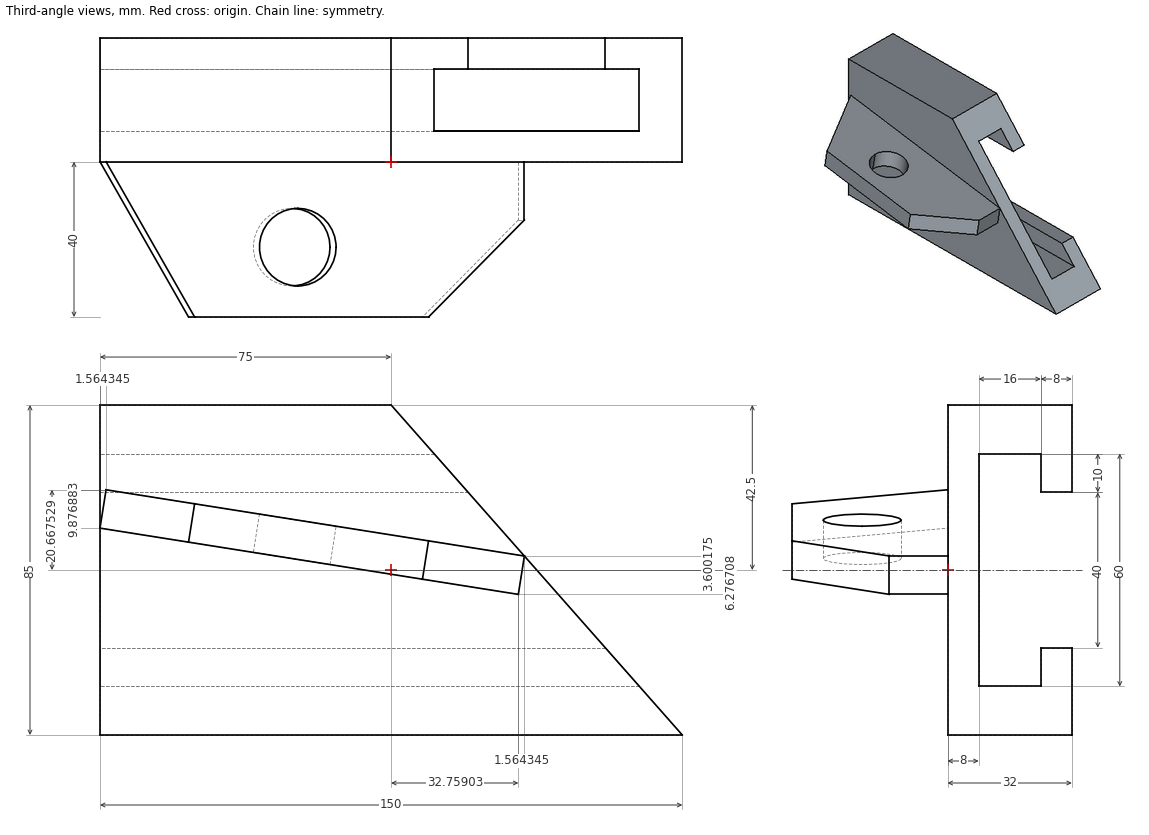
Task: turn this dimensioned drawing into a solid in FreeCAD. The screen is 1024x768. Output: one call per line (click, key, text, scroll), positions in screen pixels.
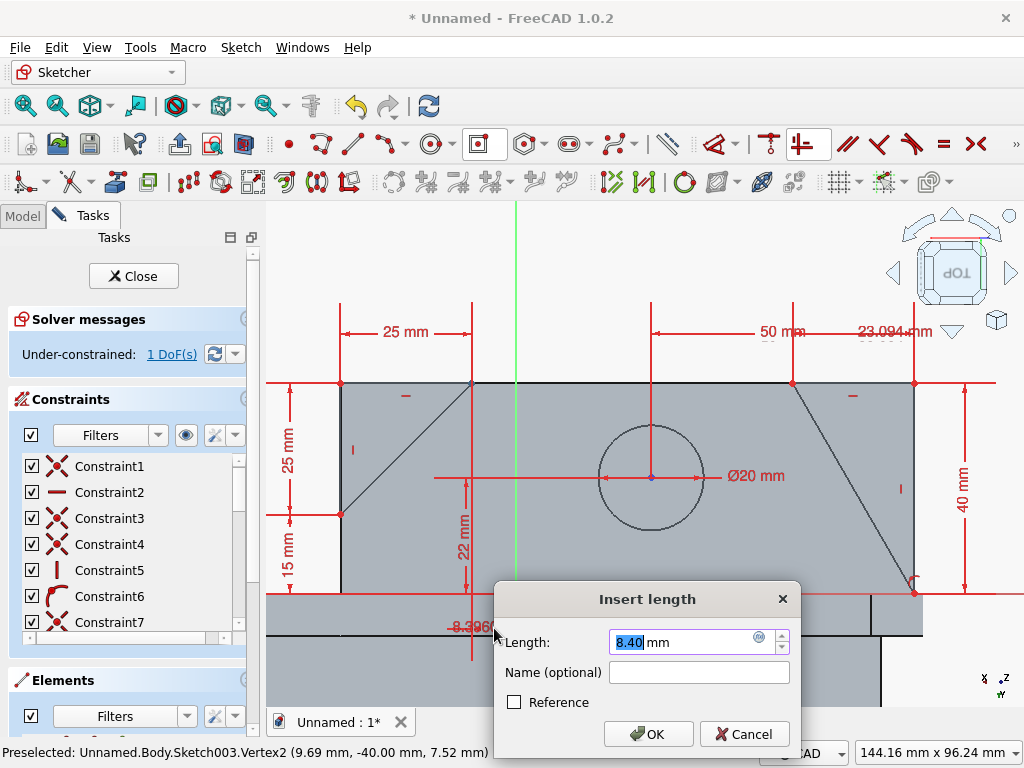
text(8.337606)
key(Return)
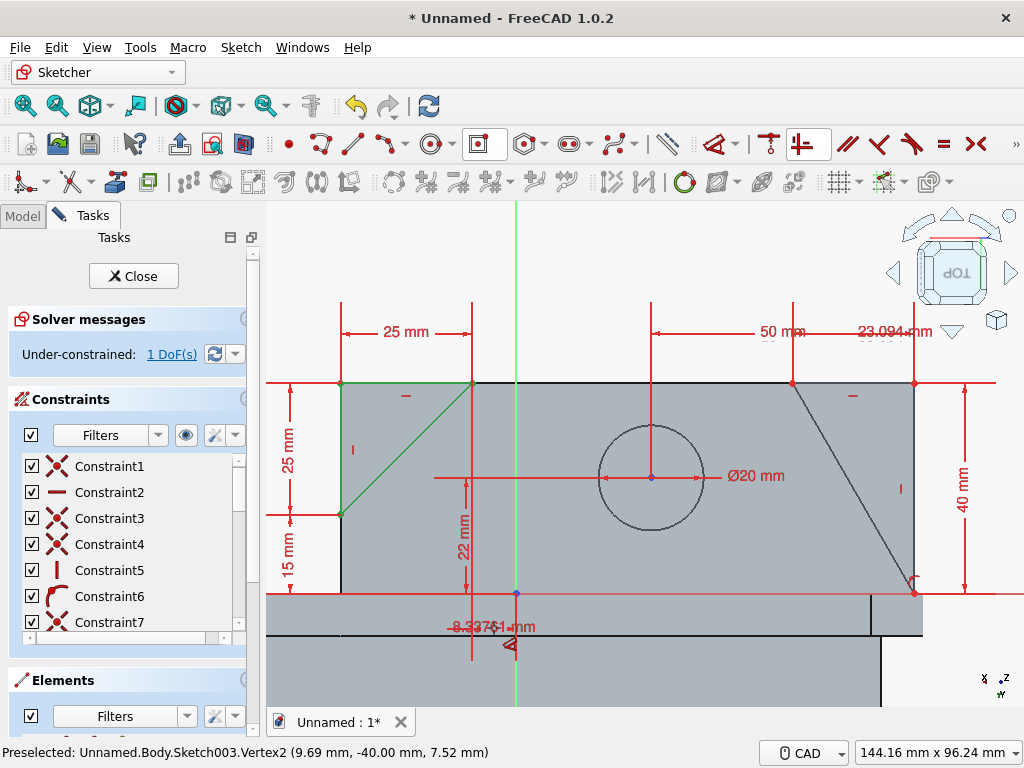
click(651, 478)
click(584, 628)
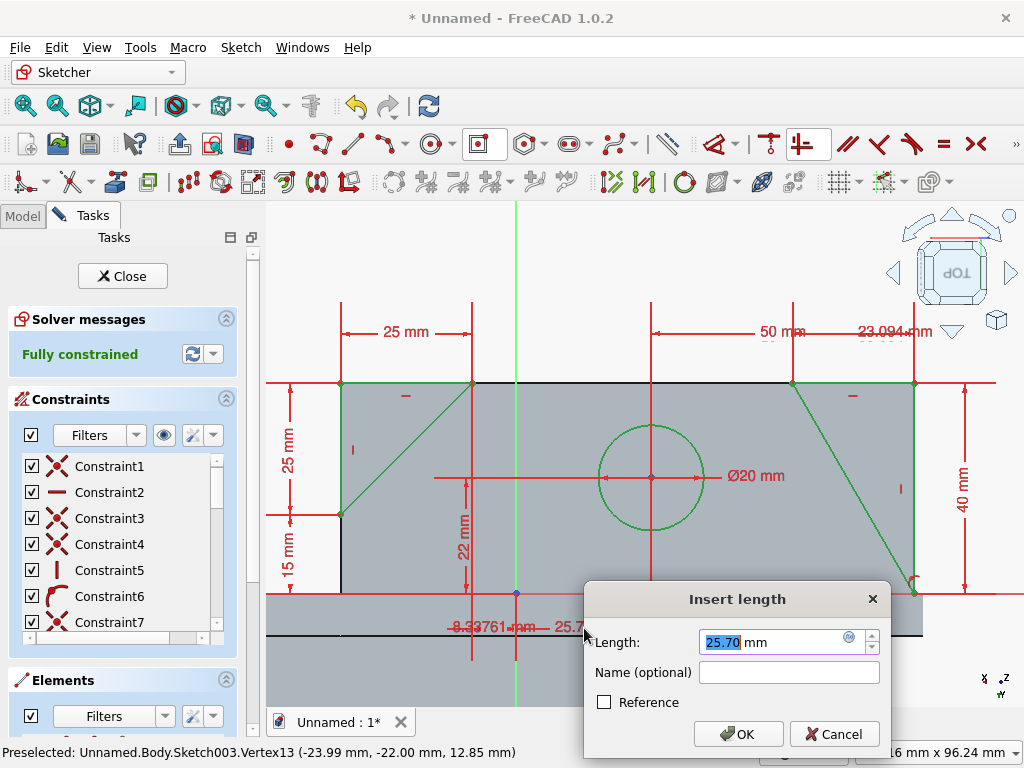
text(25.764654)
key(Return)
key(Escape)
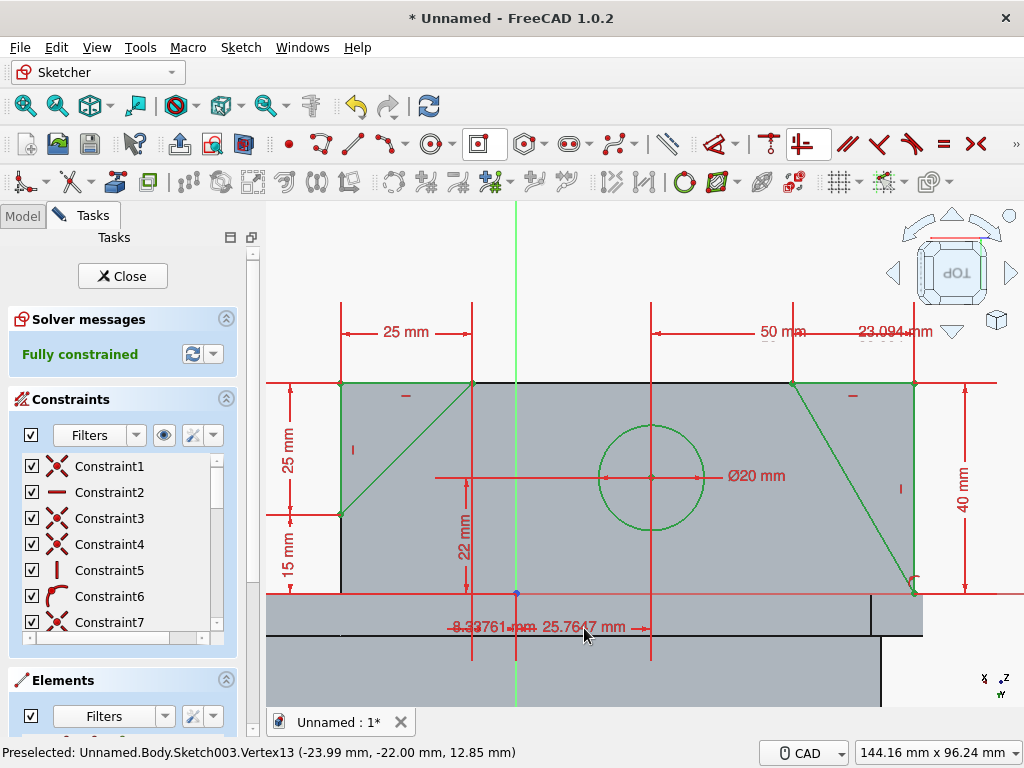
click(123, 276)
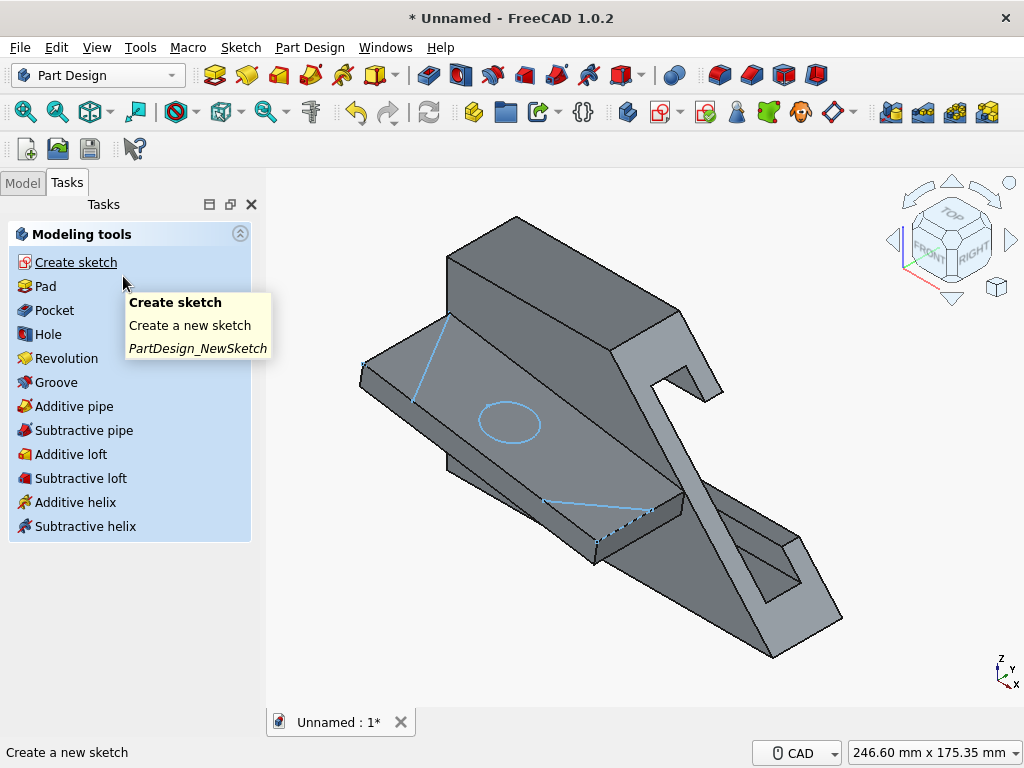
click(430, 76)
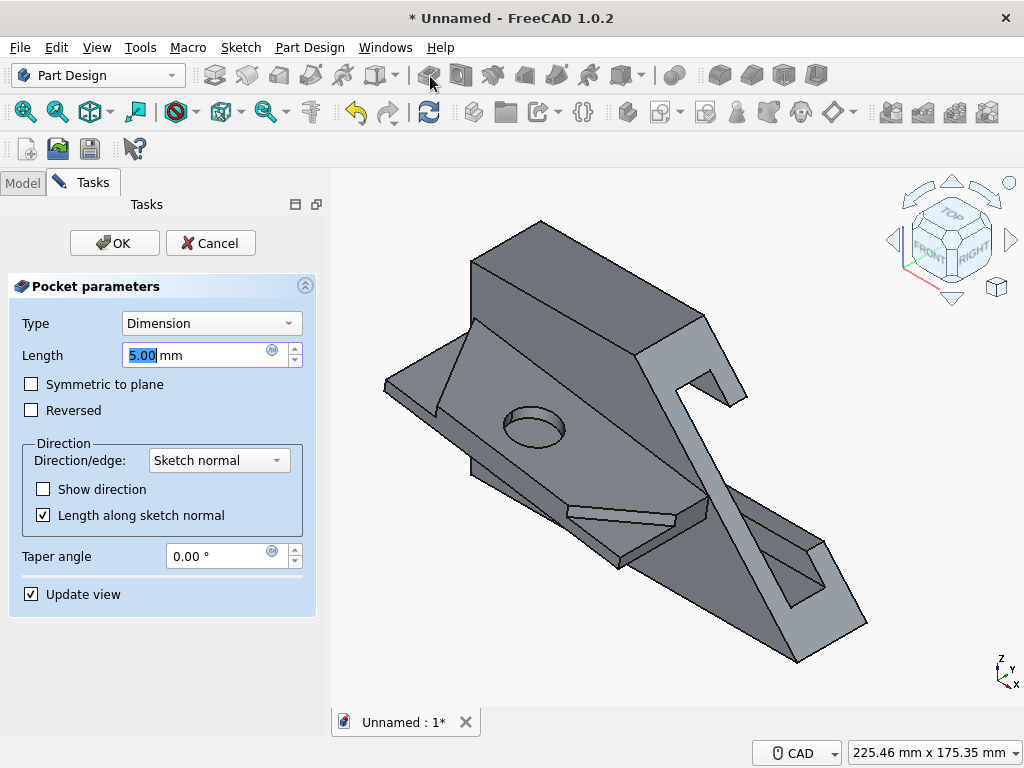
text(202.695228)
key(Tab)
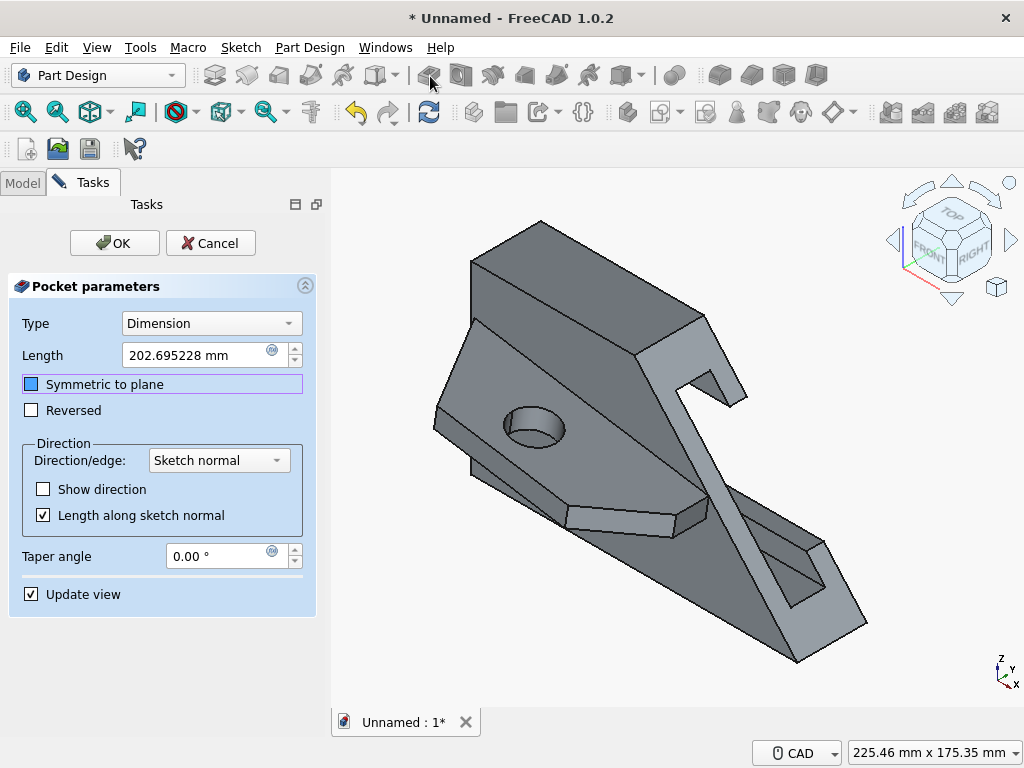
click(30, 384)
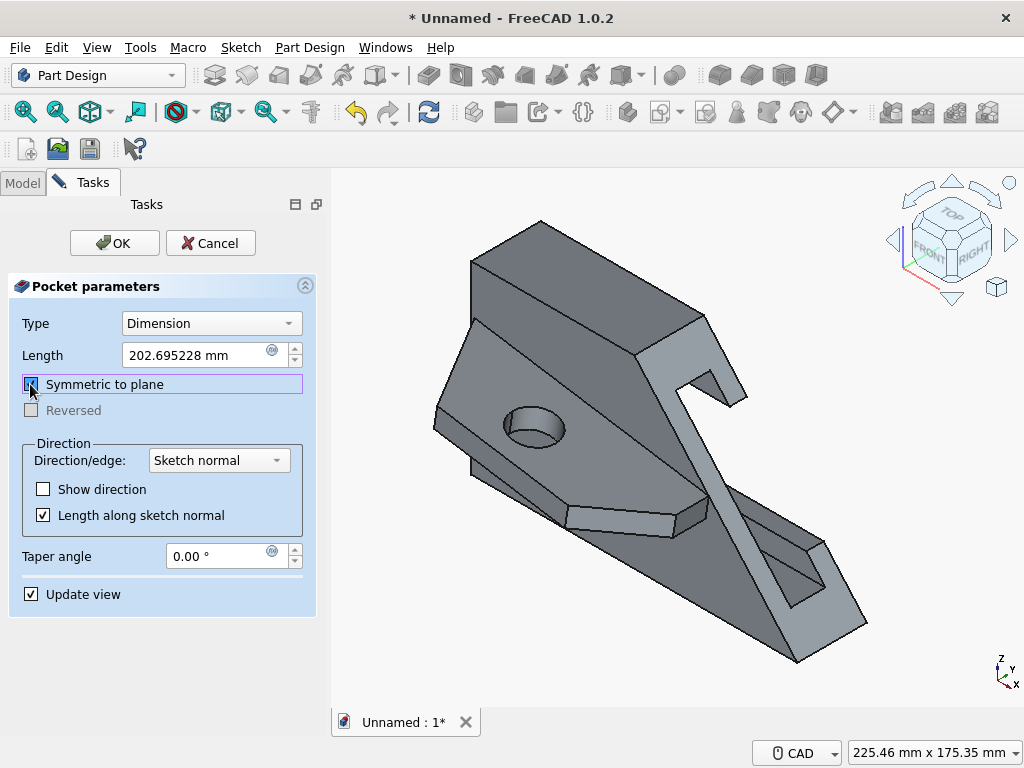
click(115, 243)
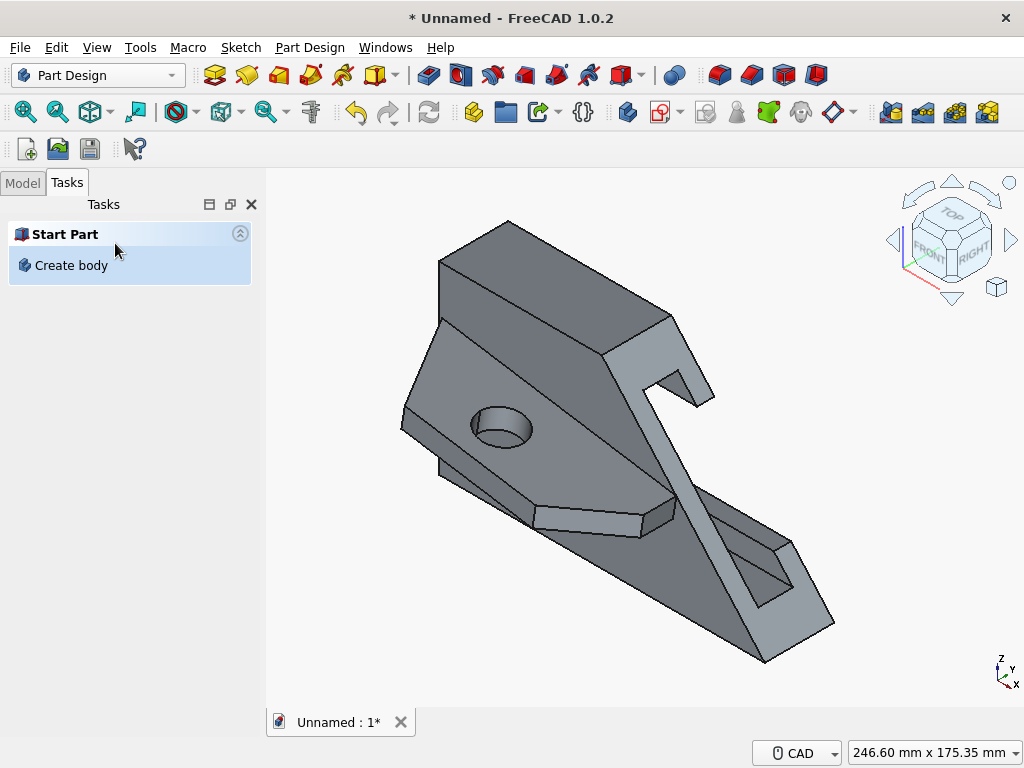
click(26, 112)